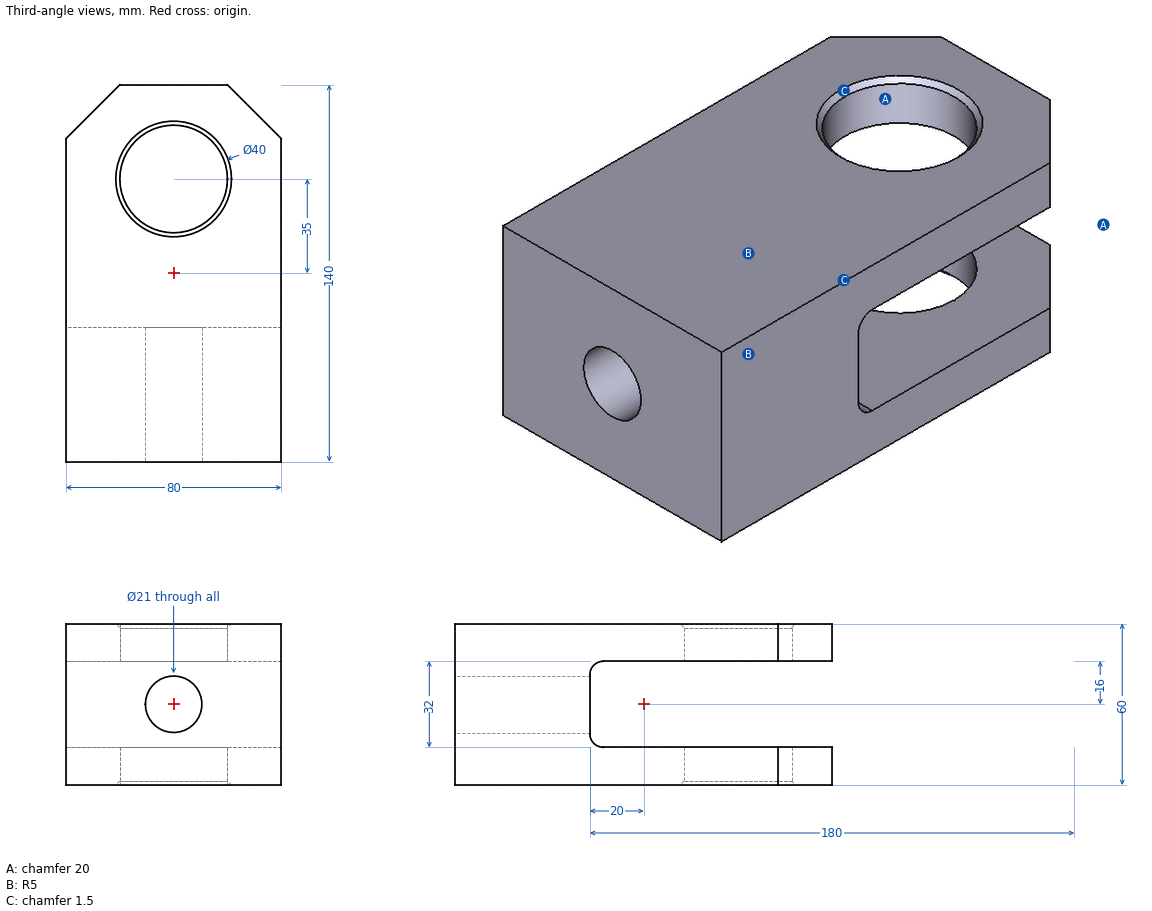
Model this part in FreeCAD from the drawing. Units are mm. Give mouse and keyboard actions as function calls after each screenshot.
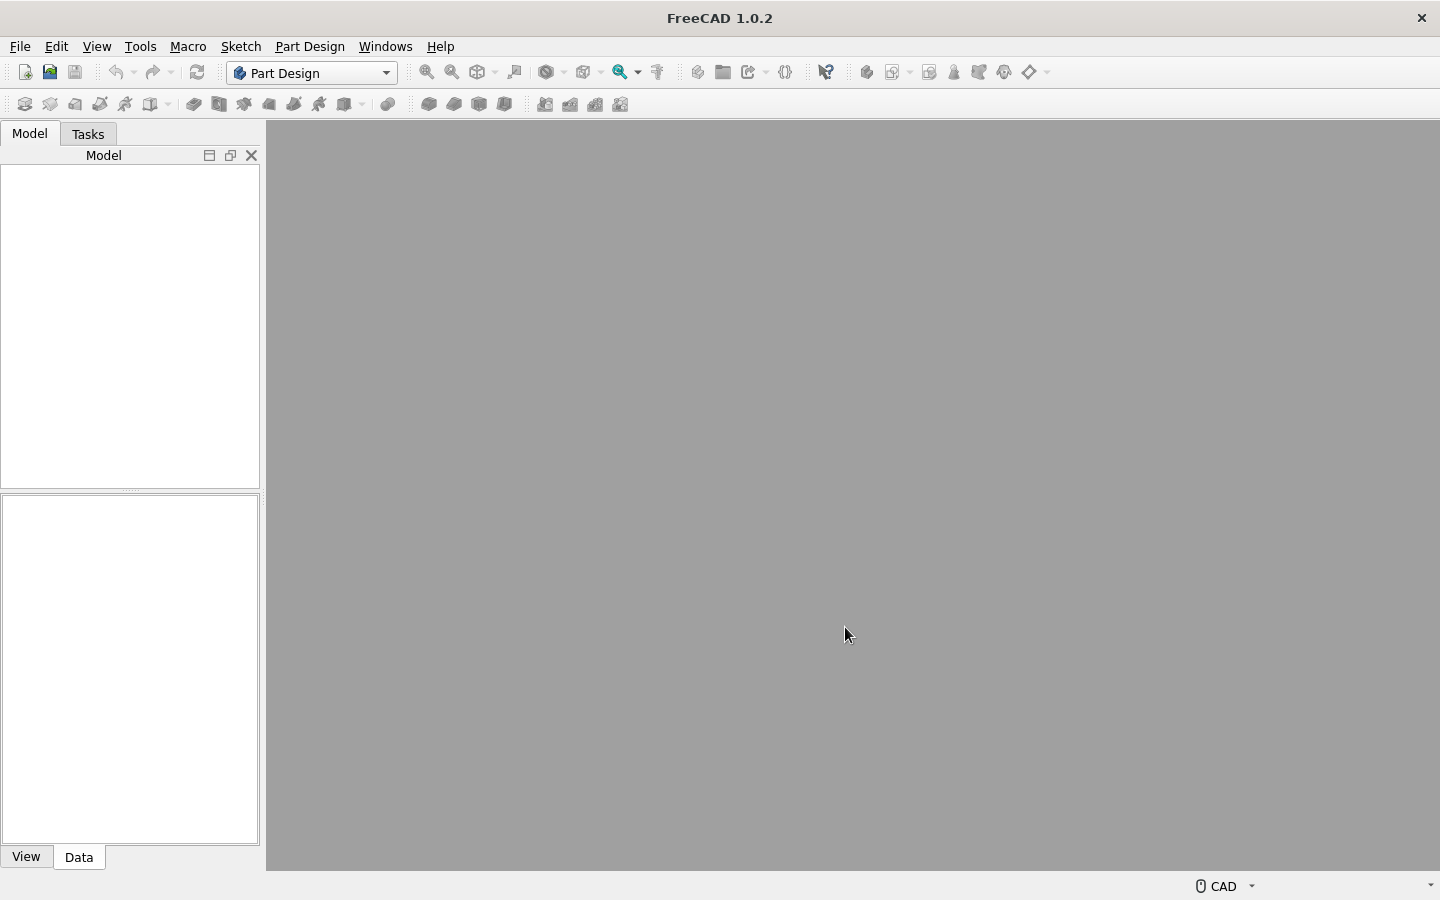
key(ctrl+n)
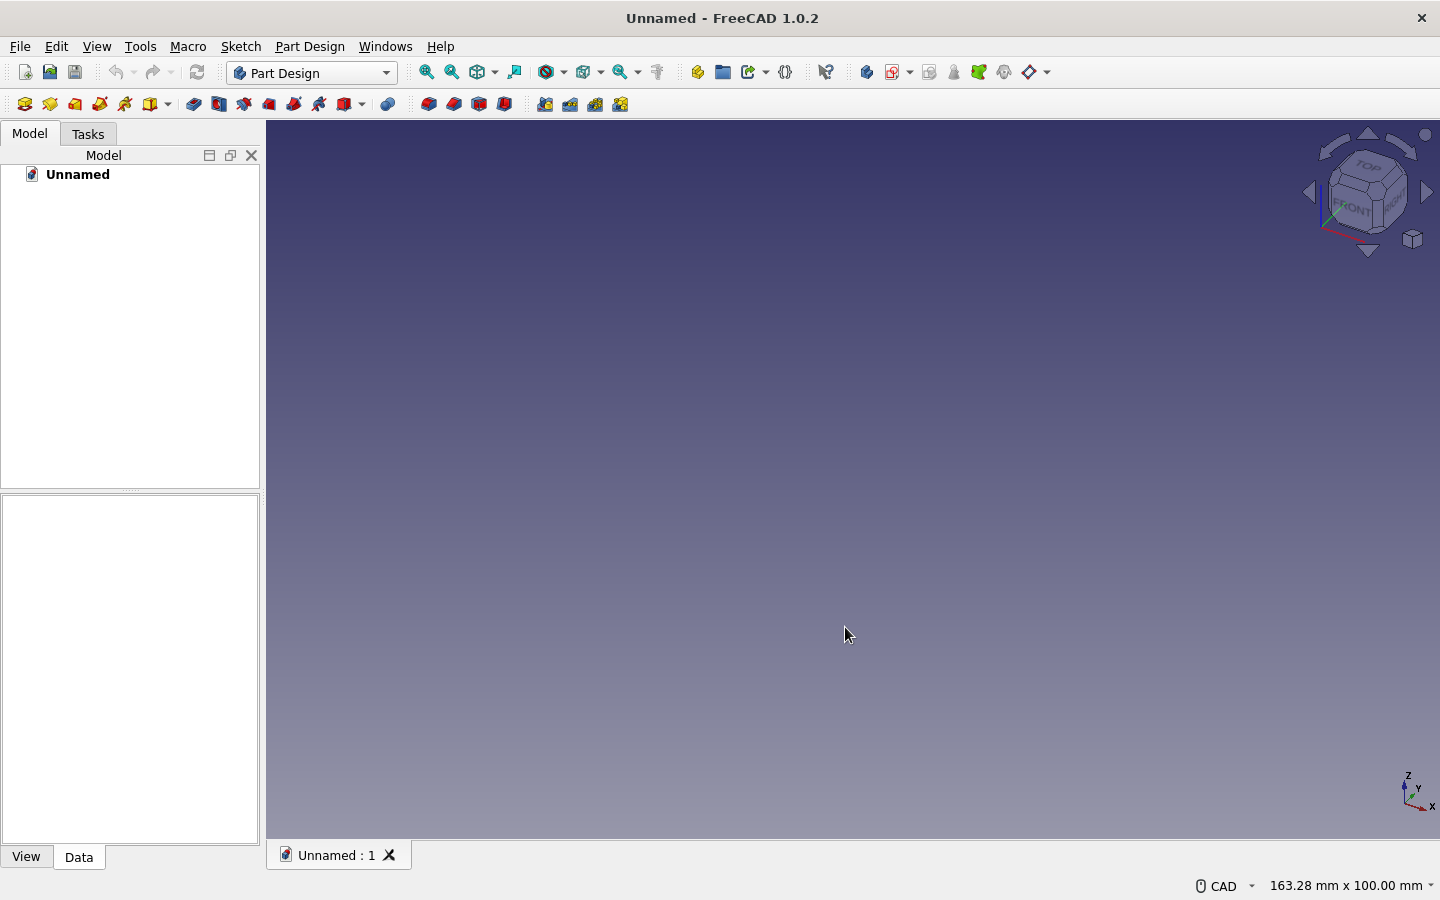
click(892, 72)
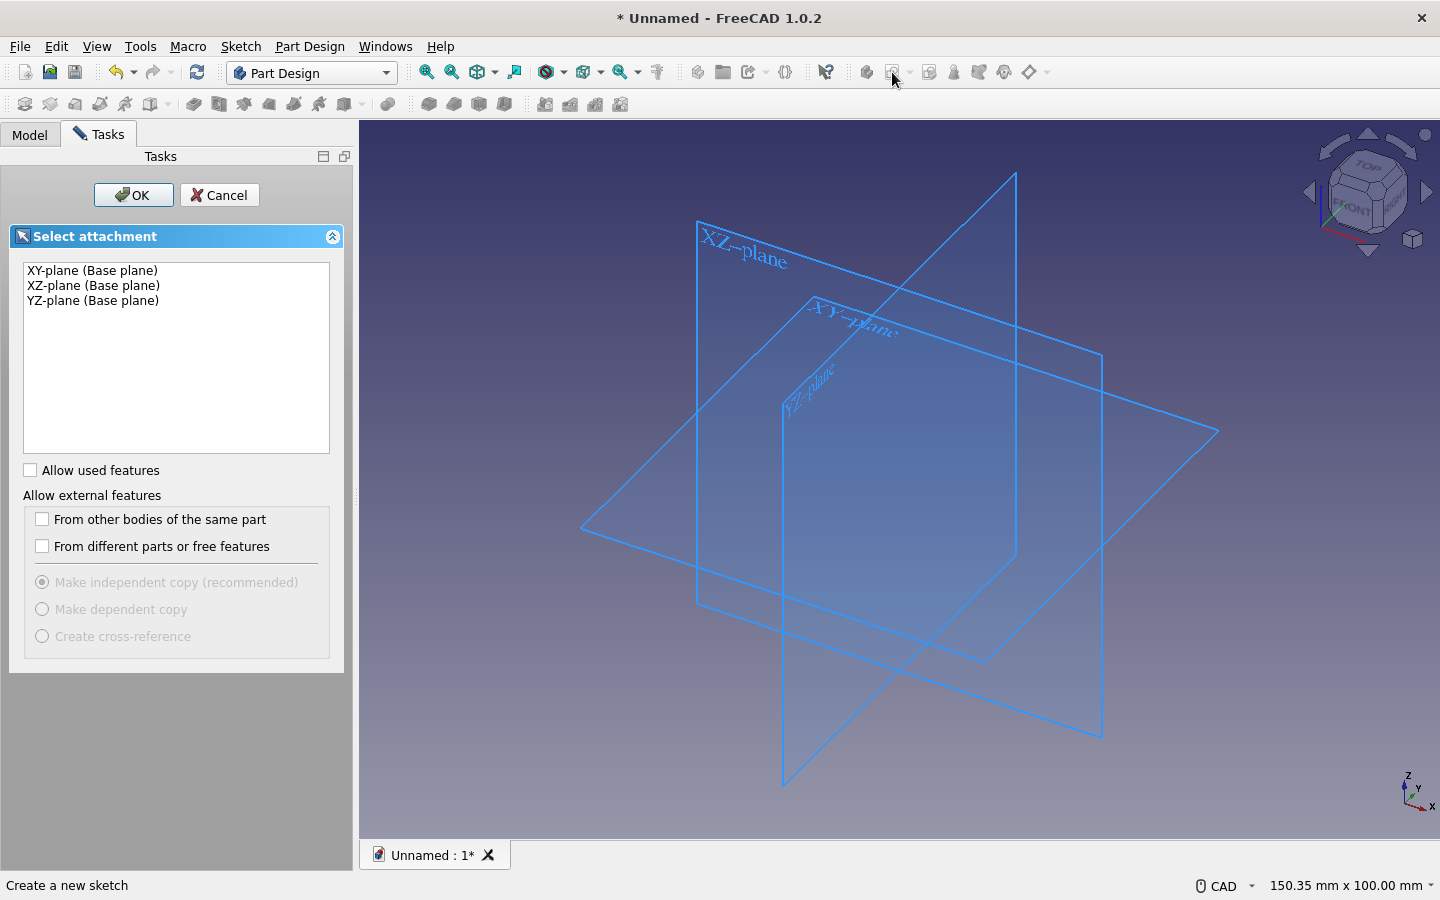
click(84, 270)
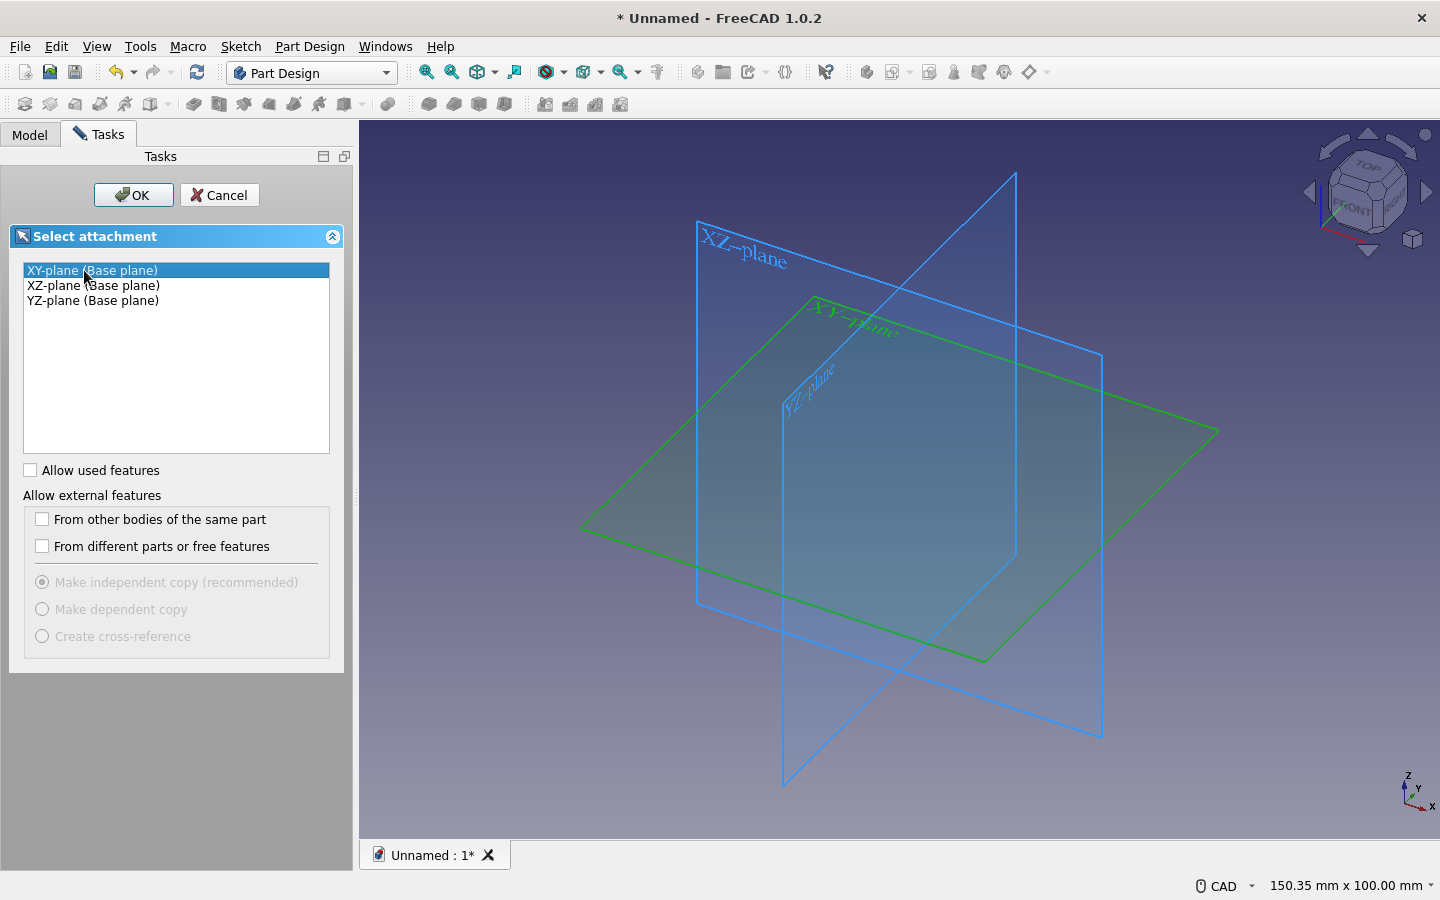
click(134, 195)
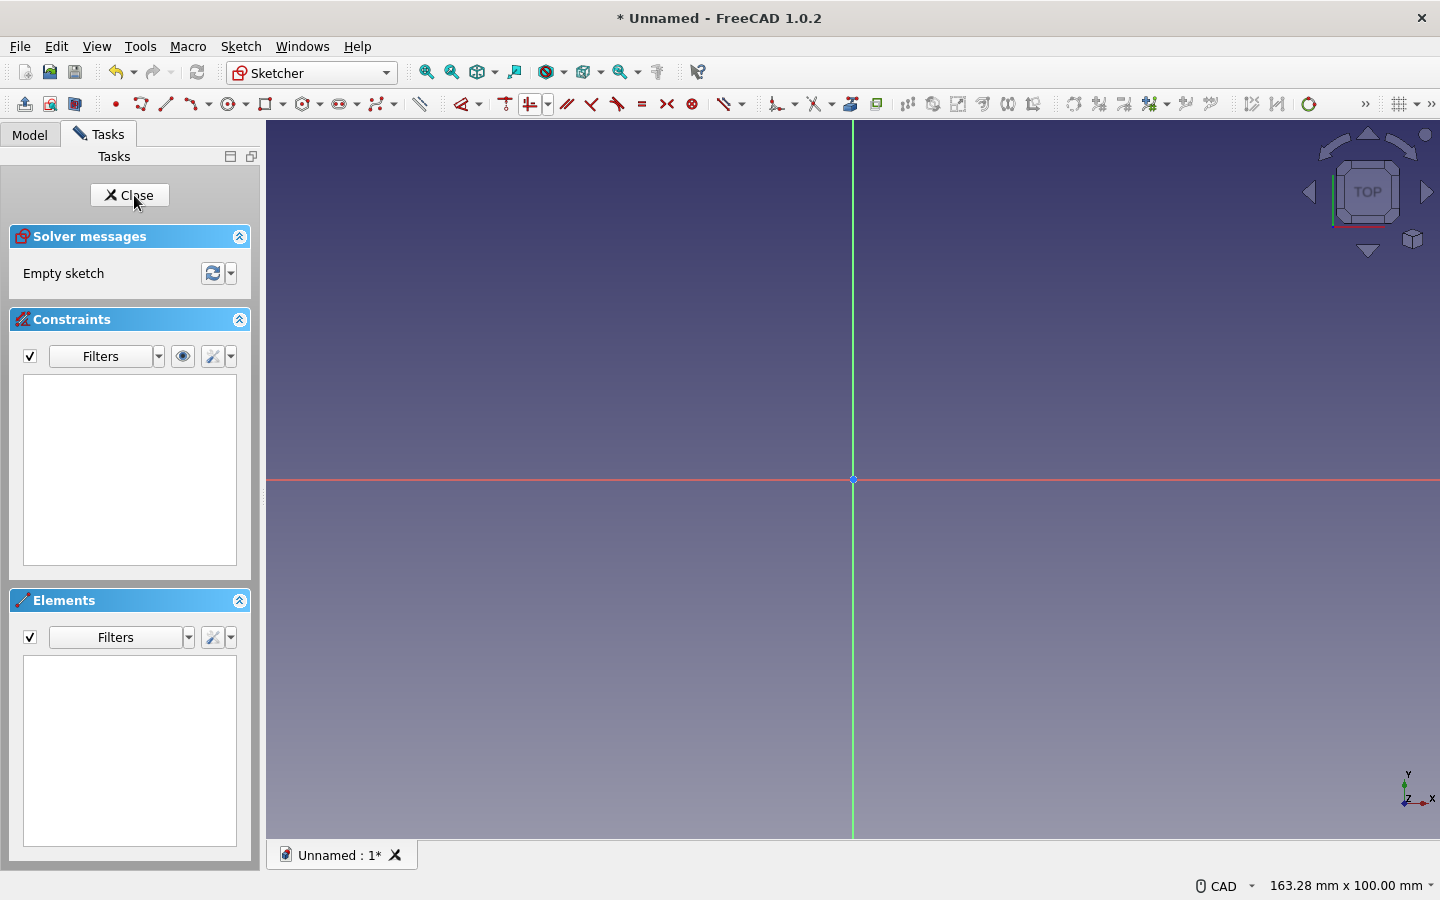
scroll(729, 480, down, 4)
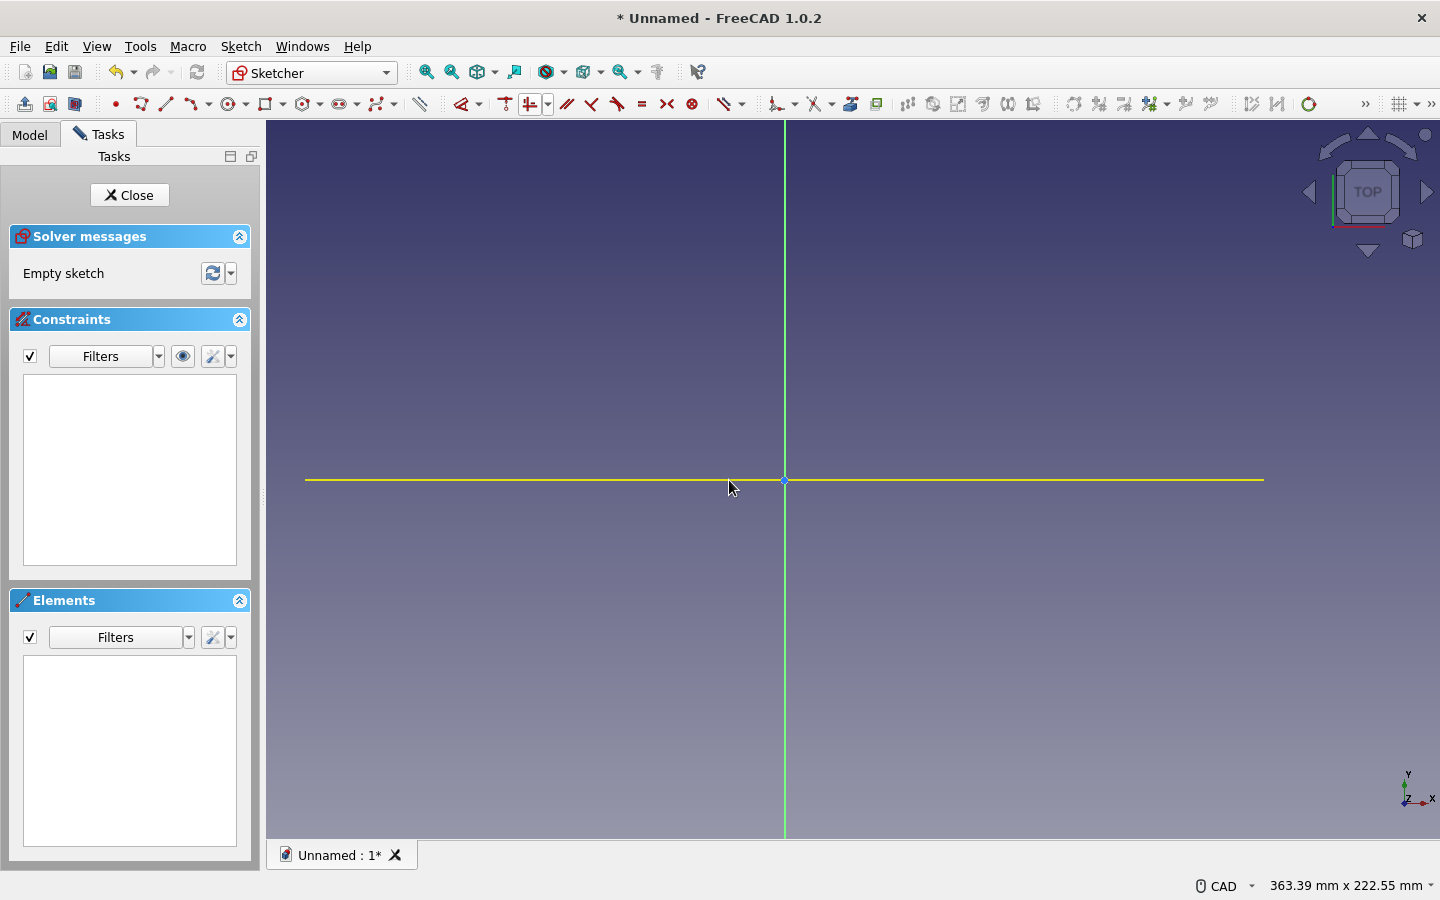
click(282, 104)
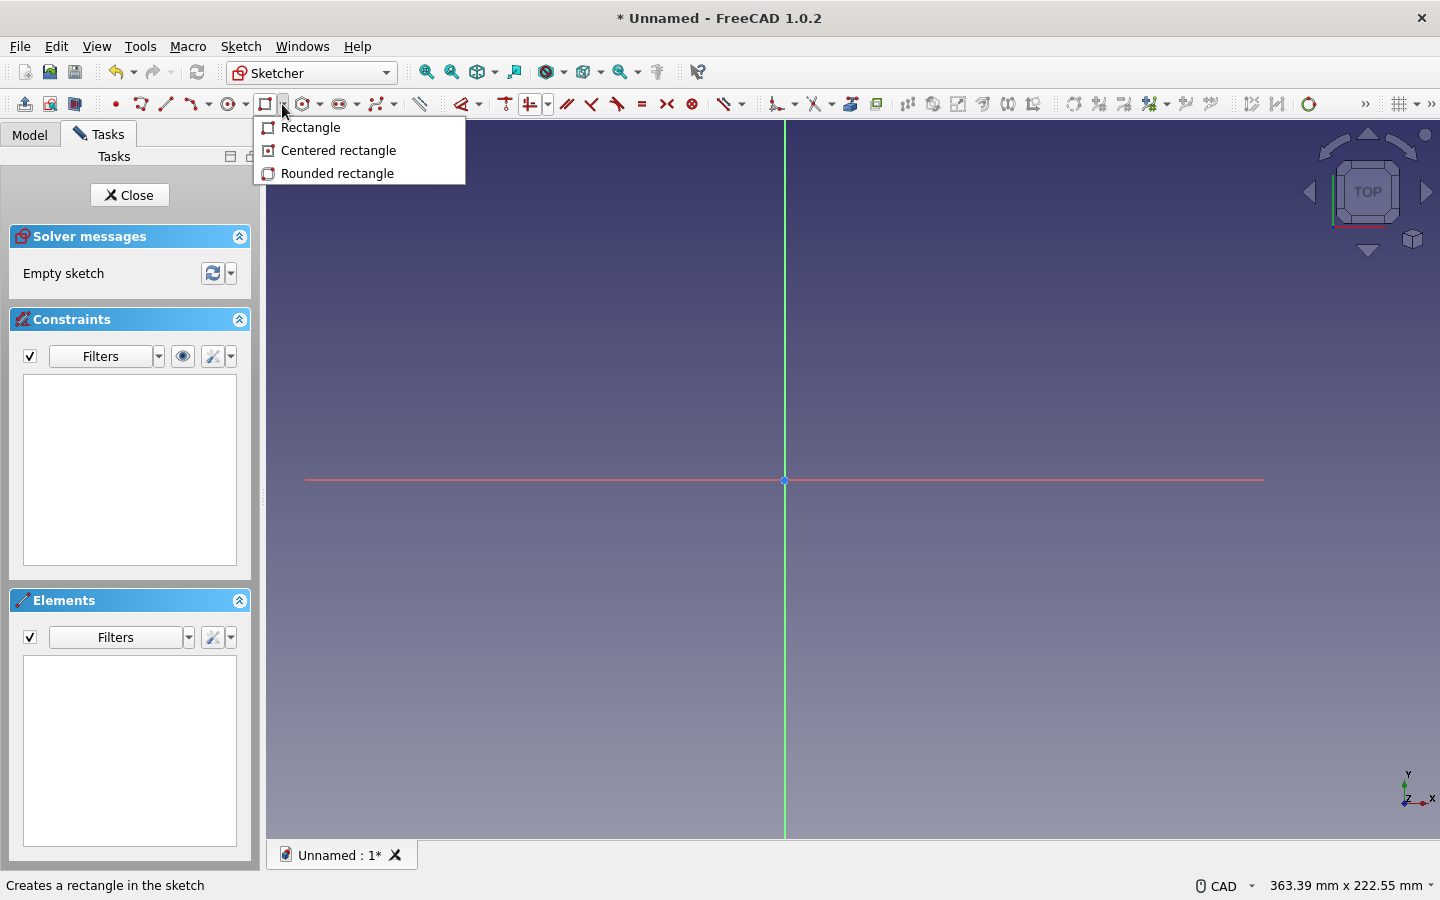
click(360, 150)